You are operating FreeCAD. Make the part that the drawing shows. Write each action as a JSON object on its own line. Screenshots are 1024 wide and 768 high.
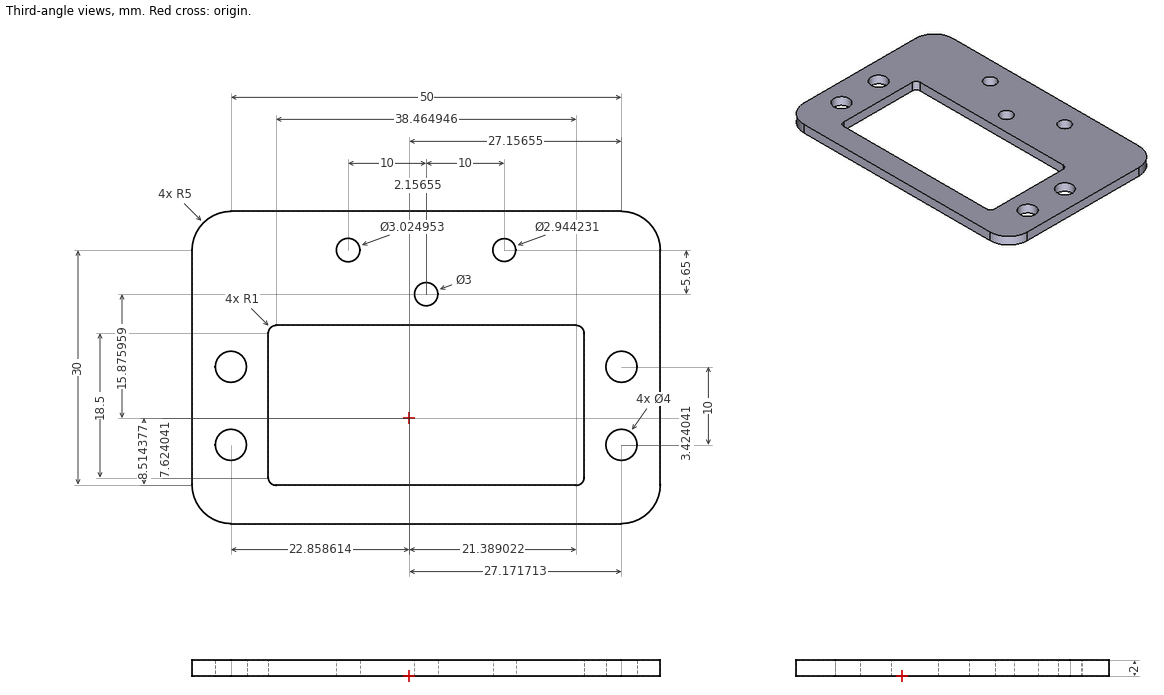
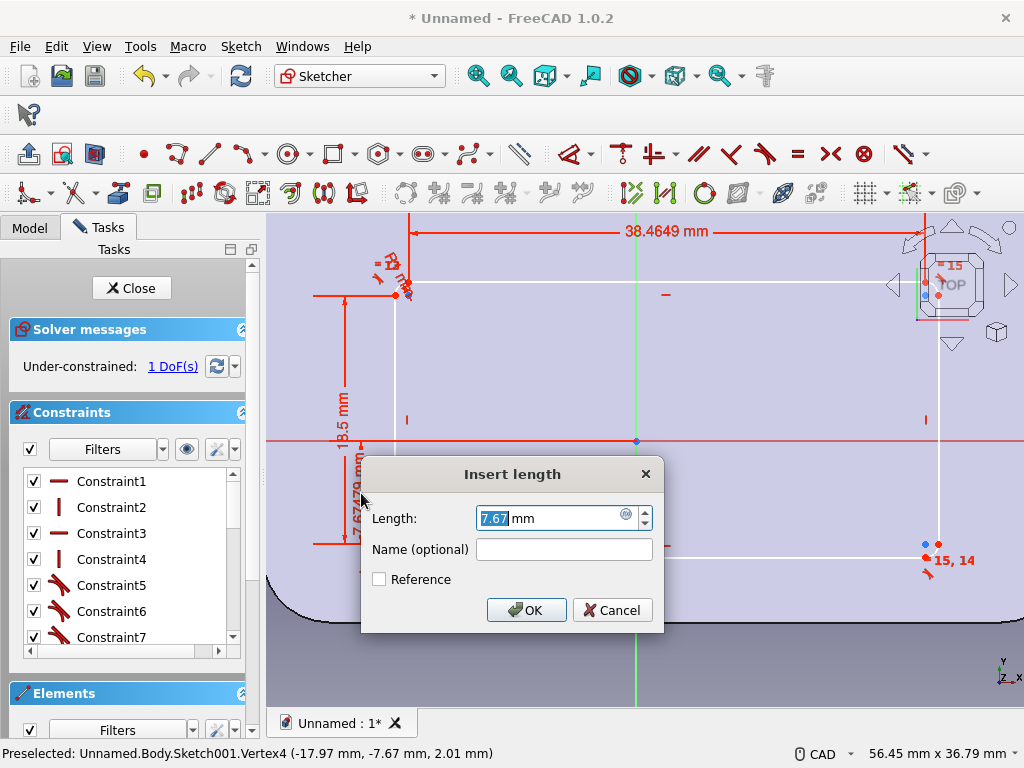
{"action": "type", "text": "7.624041"}
{"action": "key", "text": "Return"}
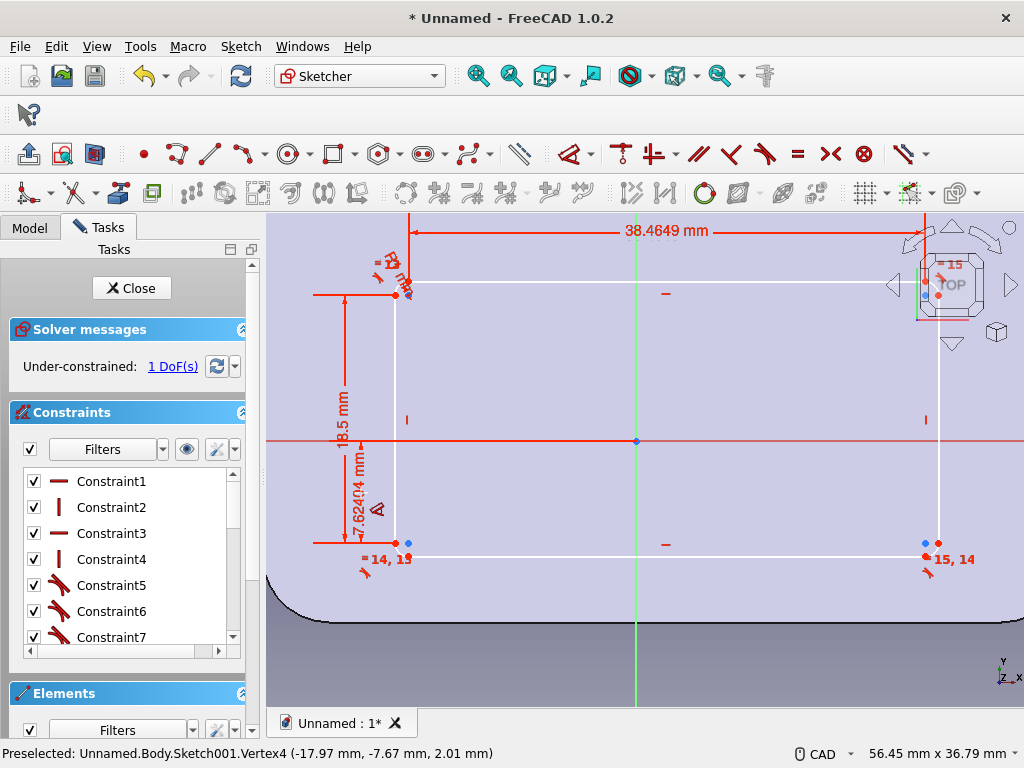
{"action": "scroll", "coordinate": [396, 543], "scroll_direction": "down", "scroll_amount": 2}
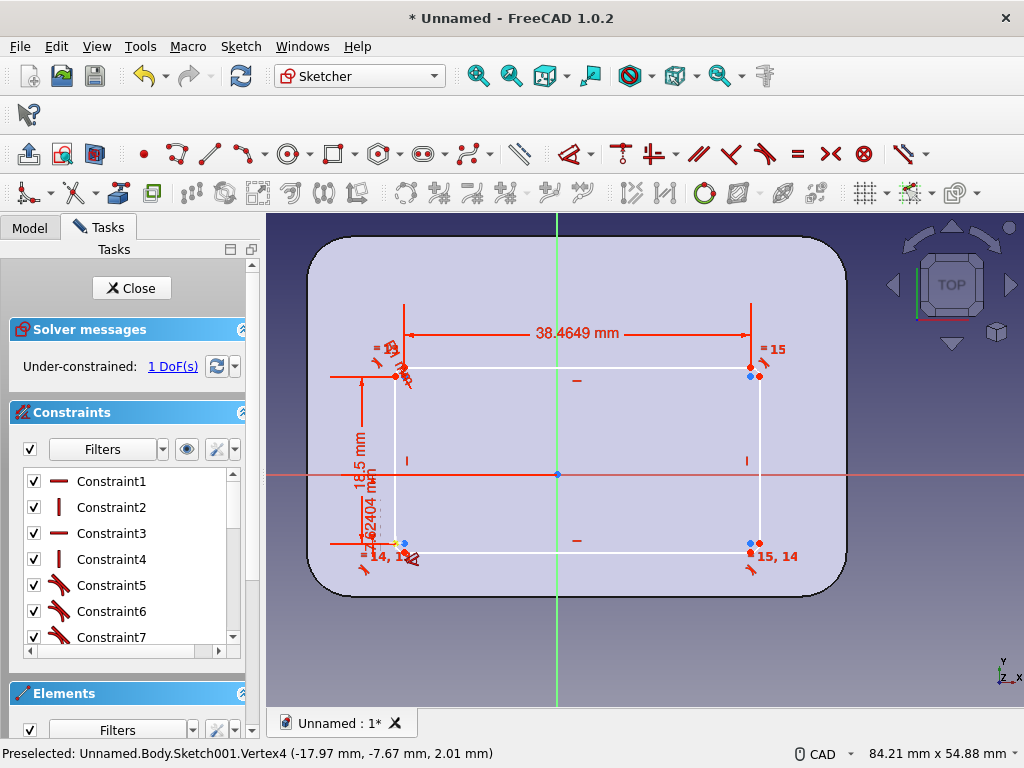
{"action": "scroll", "coordinate": [751, 368], "scroll_direction": "up", "scroll_amount": 2}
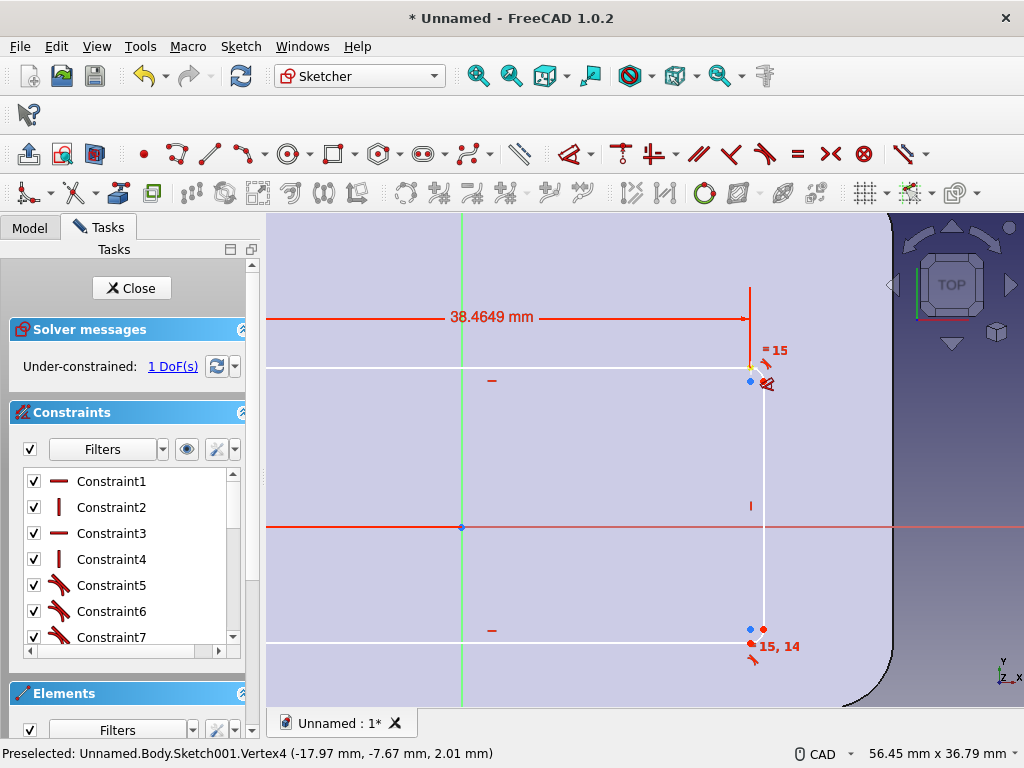
{"action": "left_click", "coordinate": [750, 368]}
{"action": "left_click", "coordinate": [606, 334]}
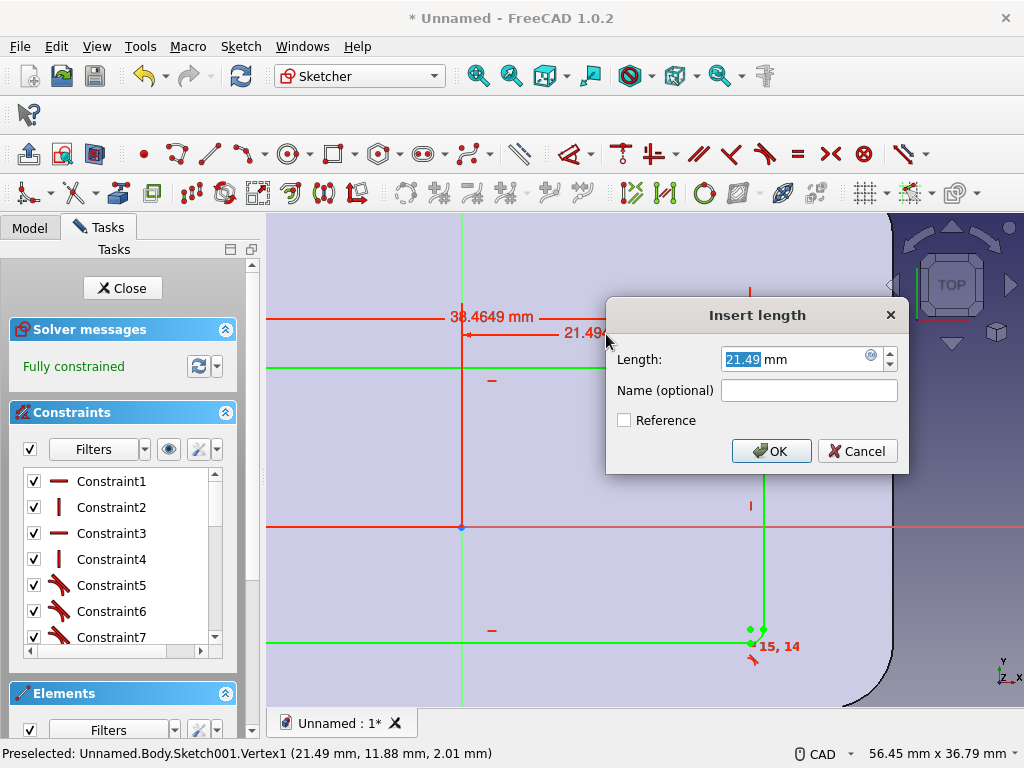
{"action": "type", "text": "21.389022"}
{"action": "key", "text": "Return"}
{"action": "key", "text": "Escape"}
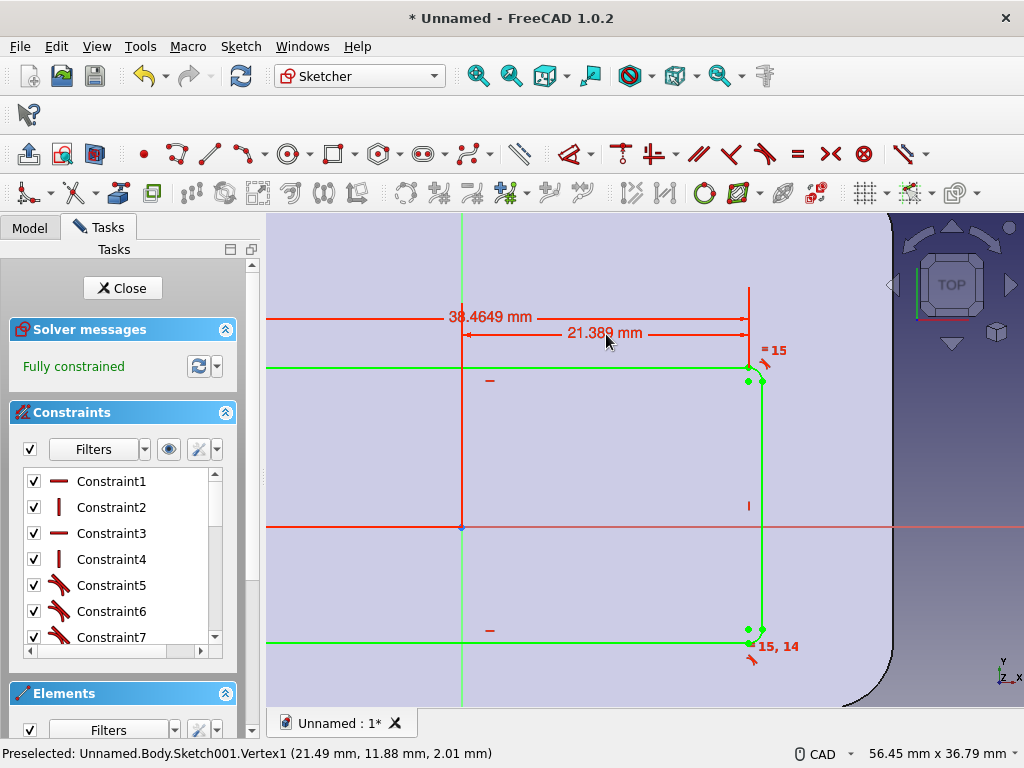
{"action": "left_click", "coordinate": [123, 288]}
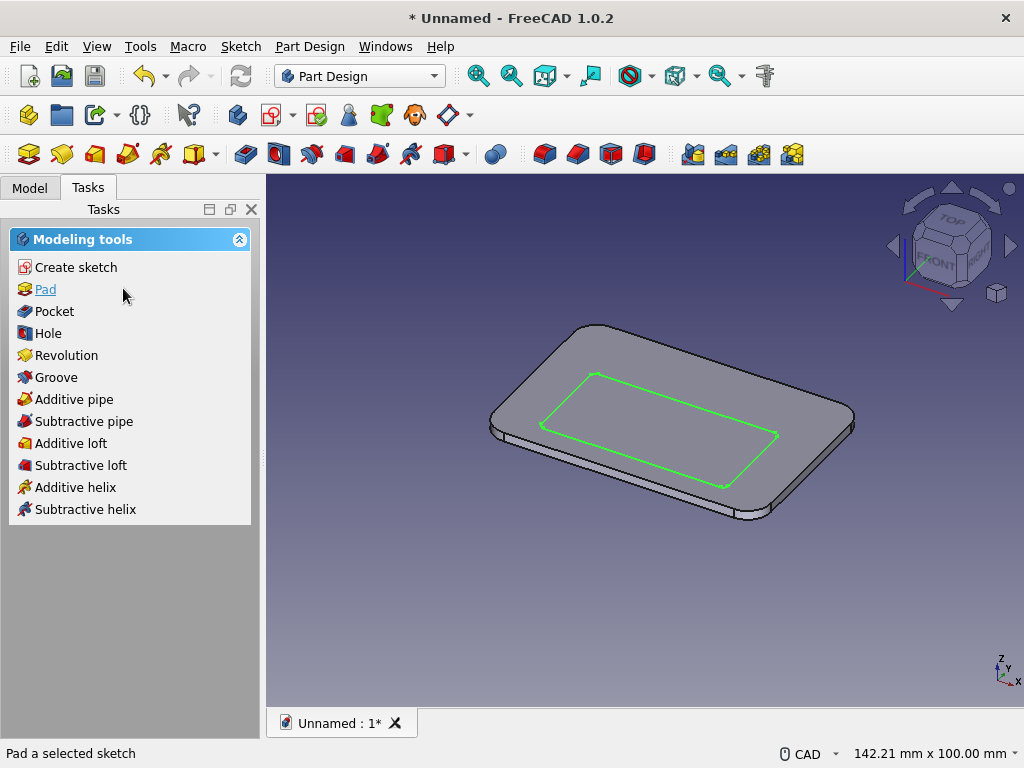
{"action": "left_click", "coordinate": [246, 154]}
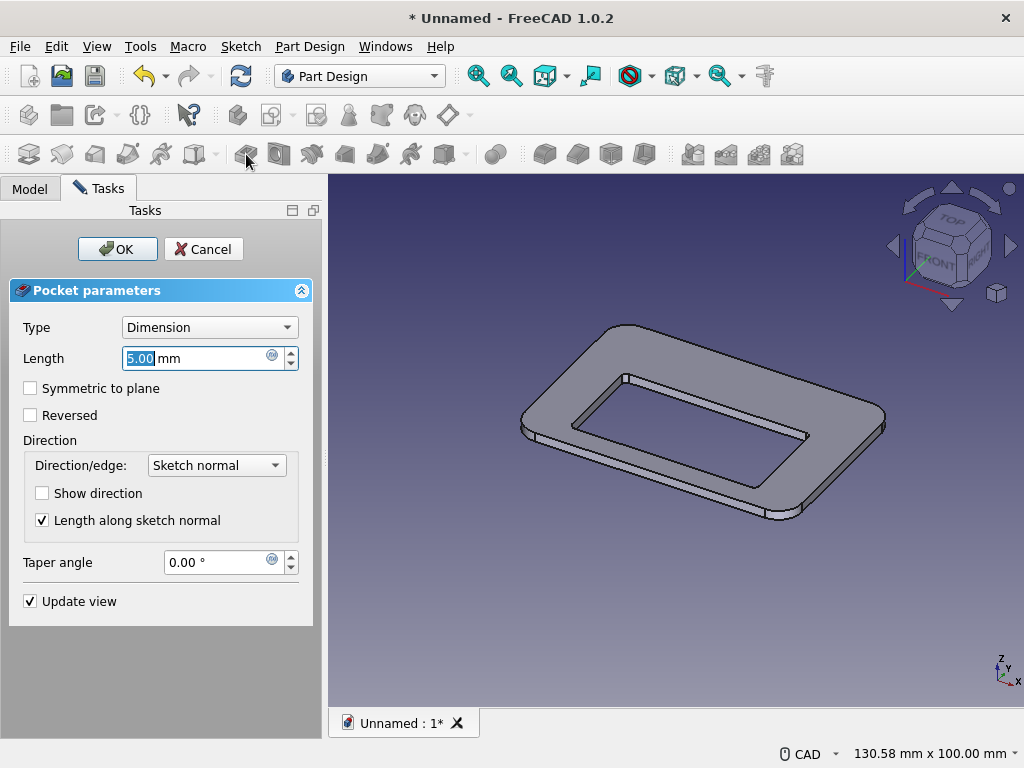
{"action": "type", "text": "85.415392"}
{"action": "key", "text": "Tab"}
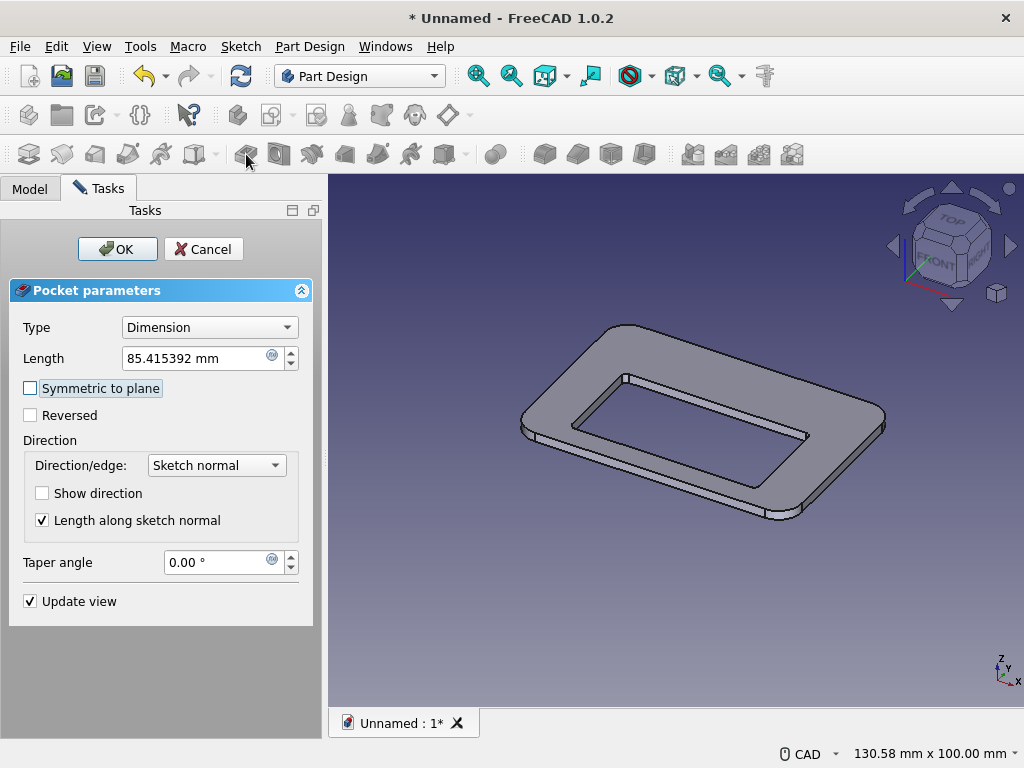
{"action": "left_click", "coordinate": [31, 388]}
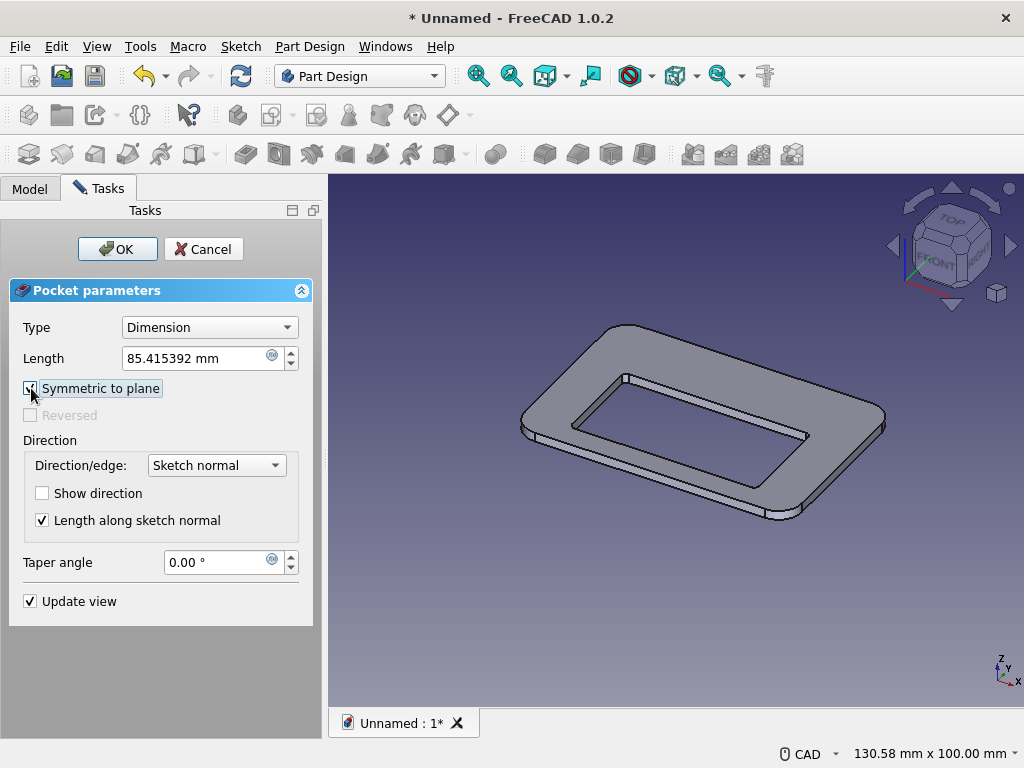
{"action": "left_click", "coordinate": [118, 249]}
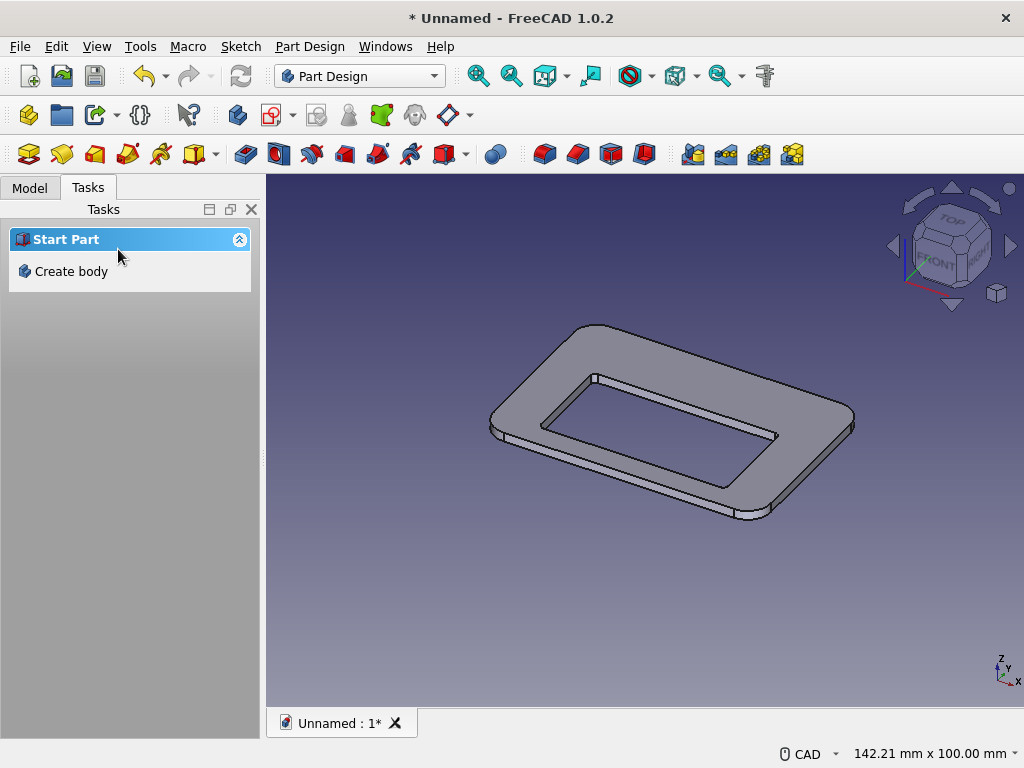
{"action": "left_click", "coordinate": [782, 413]}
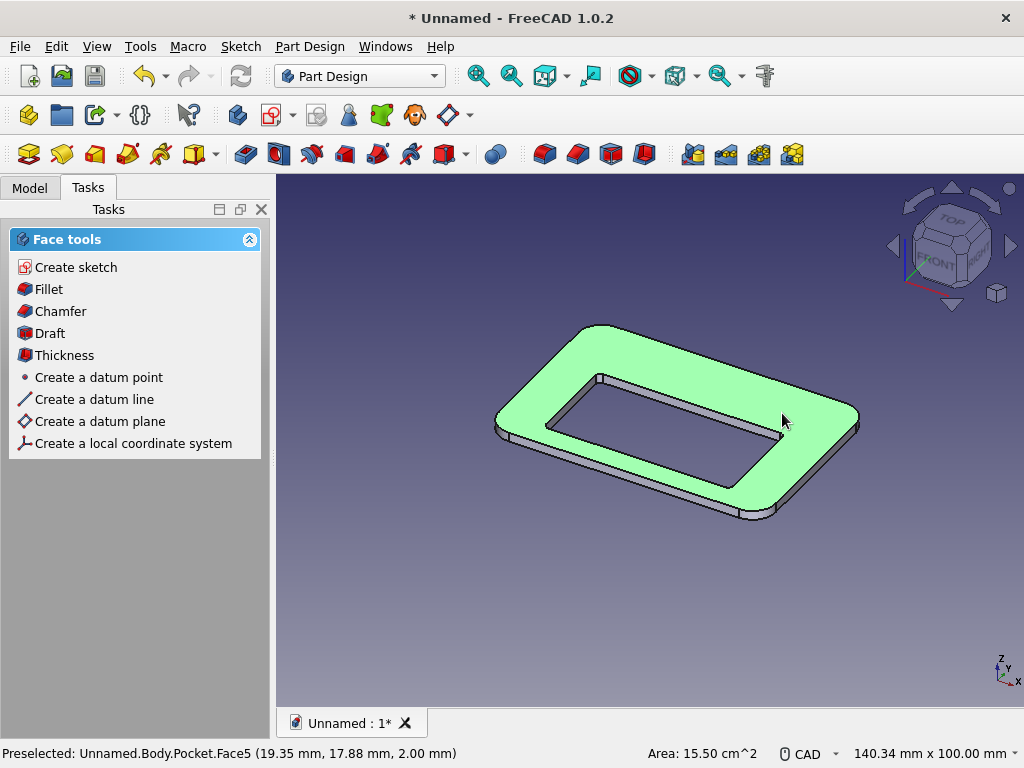
{"action": "left_click", "coordinate": [270, 116]}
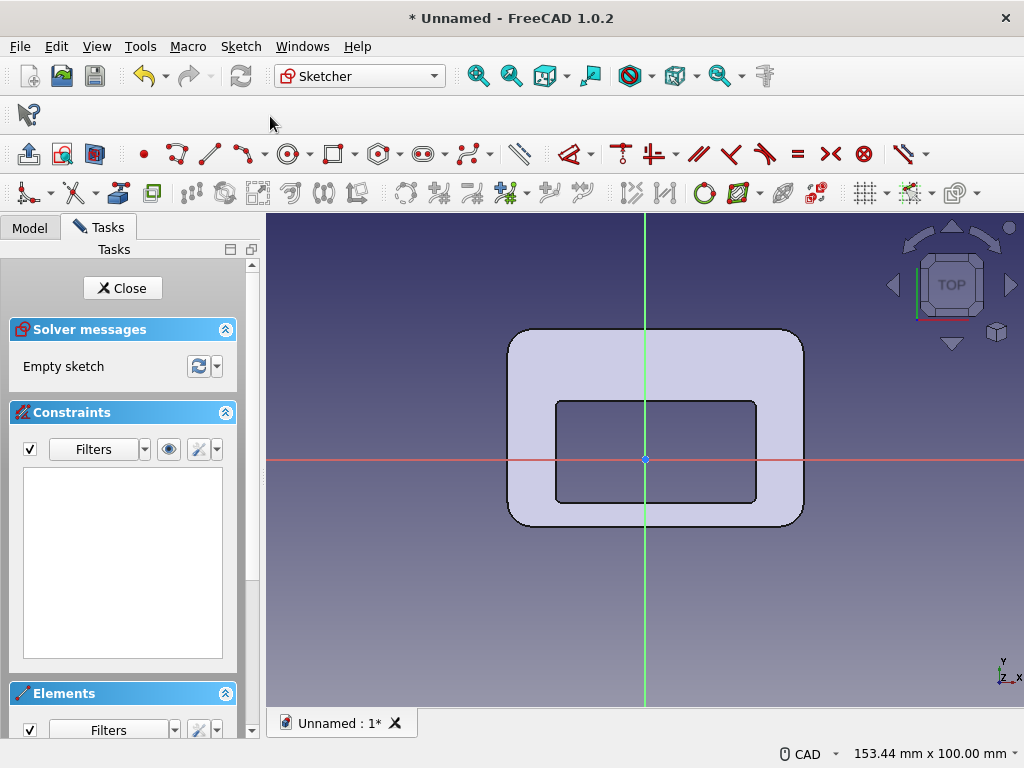
{"action": "scroll", "coordinate": [702, 370], "scroll_direction": "up", "scroll_amount": 5}